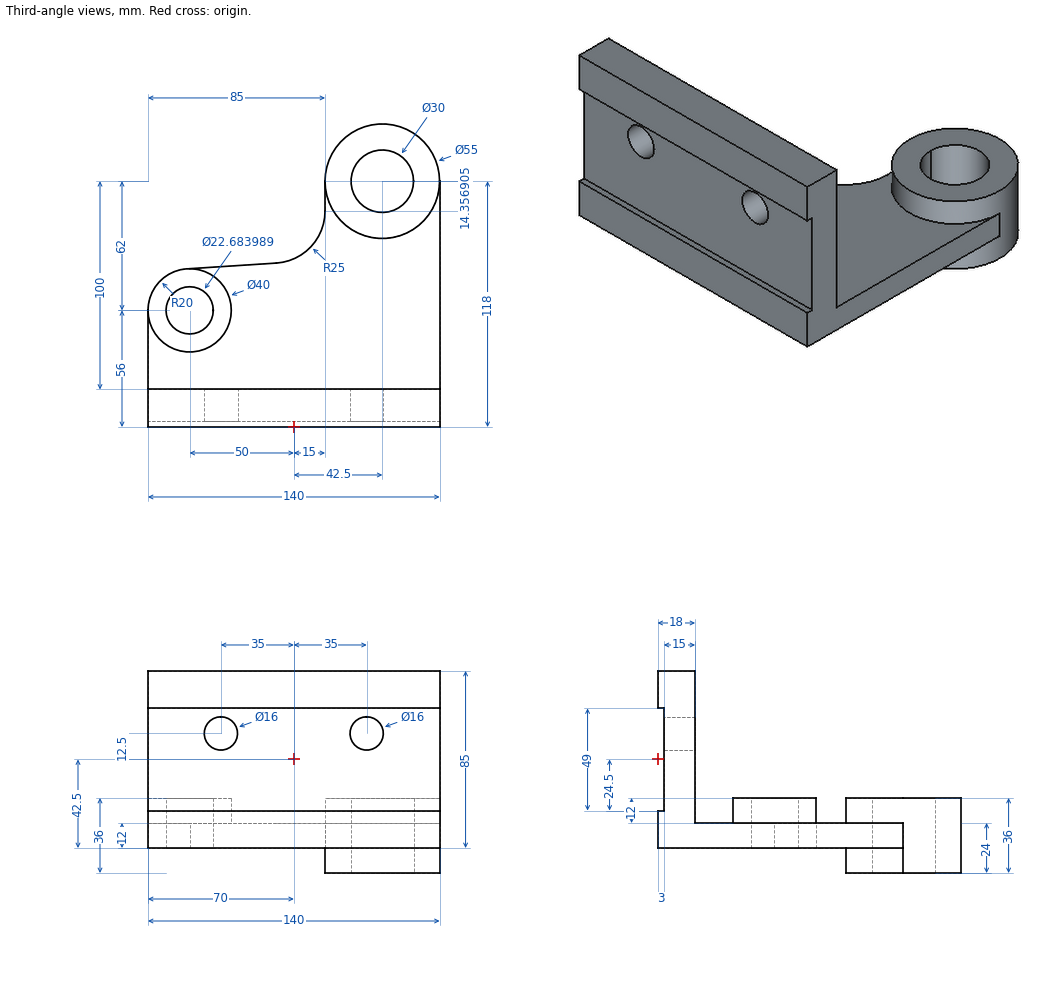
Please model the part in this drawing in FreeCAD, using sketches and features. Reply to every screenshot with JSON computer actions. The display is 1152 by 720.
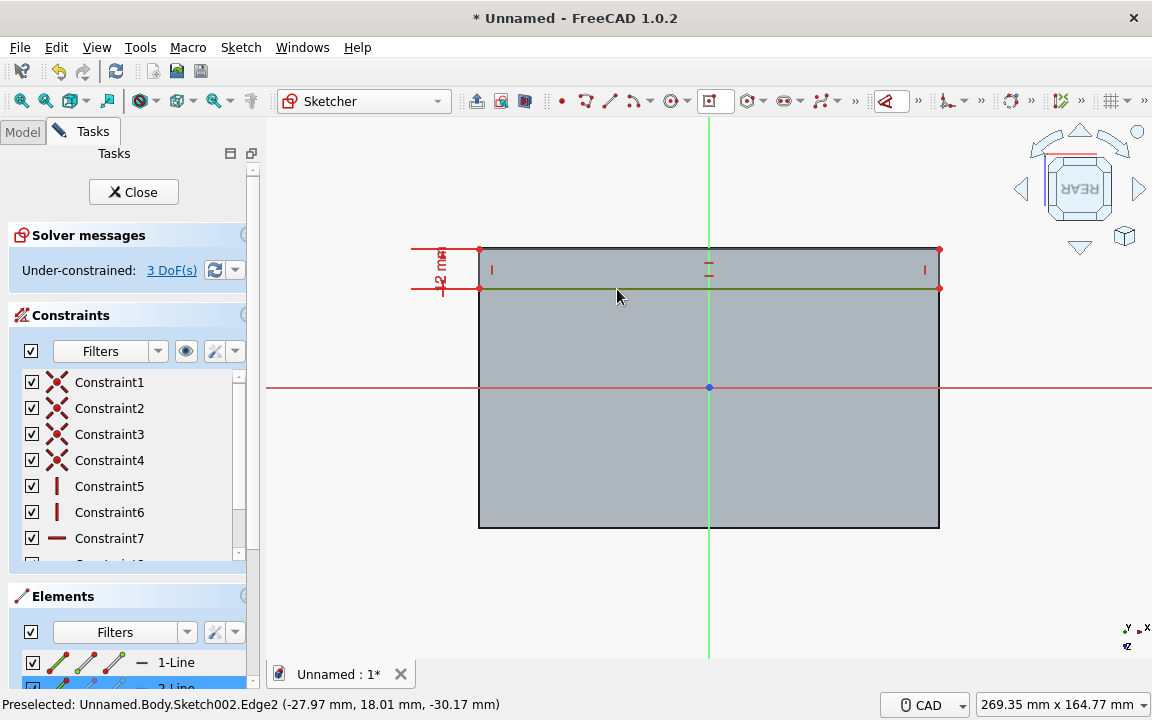
{"action": "key", "text": "l"}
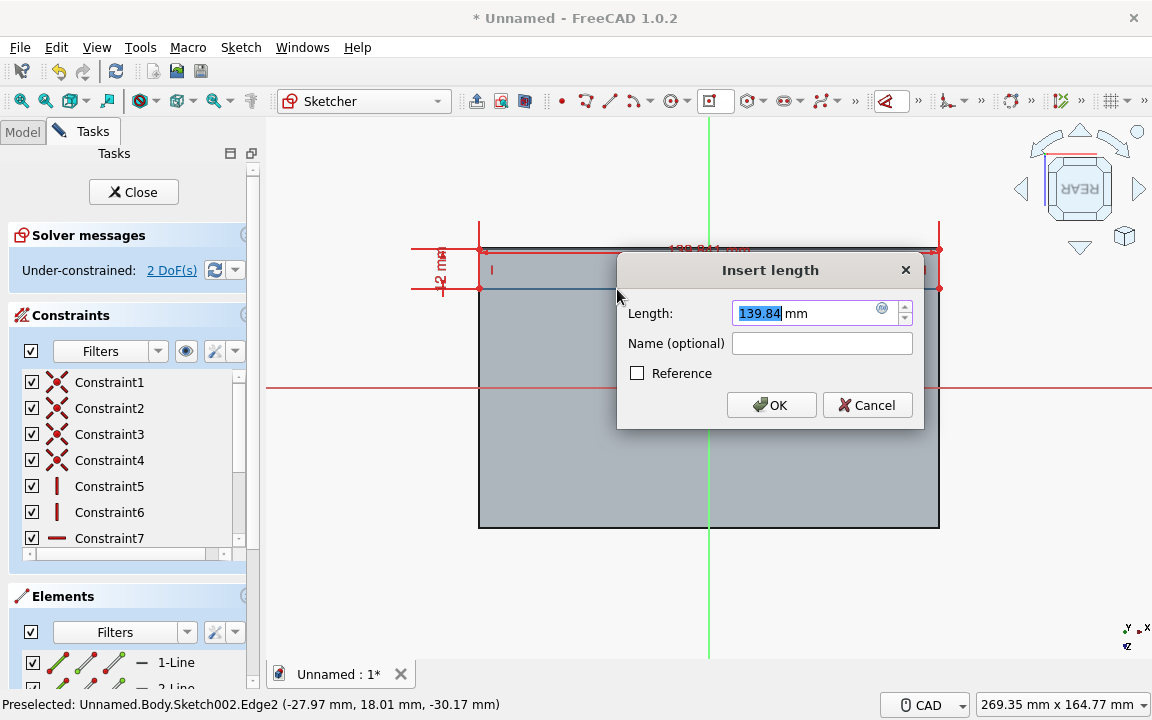
{"action": "type", "text": "140"}
{"action": "key", "text": "Return"}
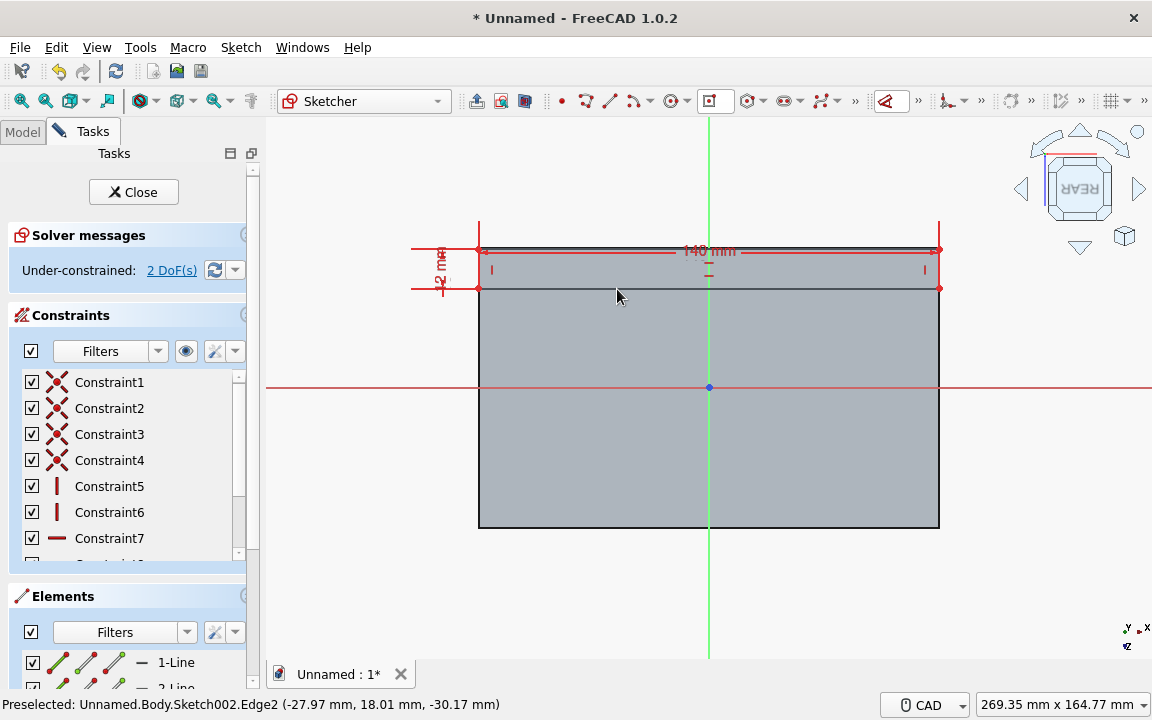
{"action": "left_click", "coordinate": [479, 249]}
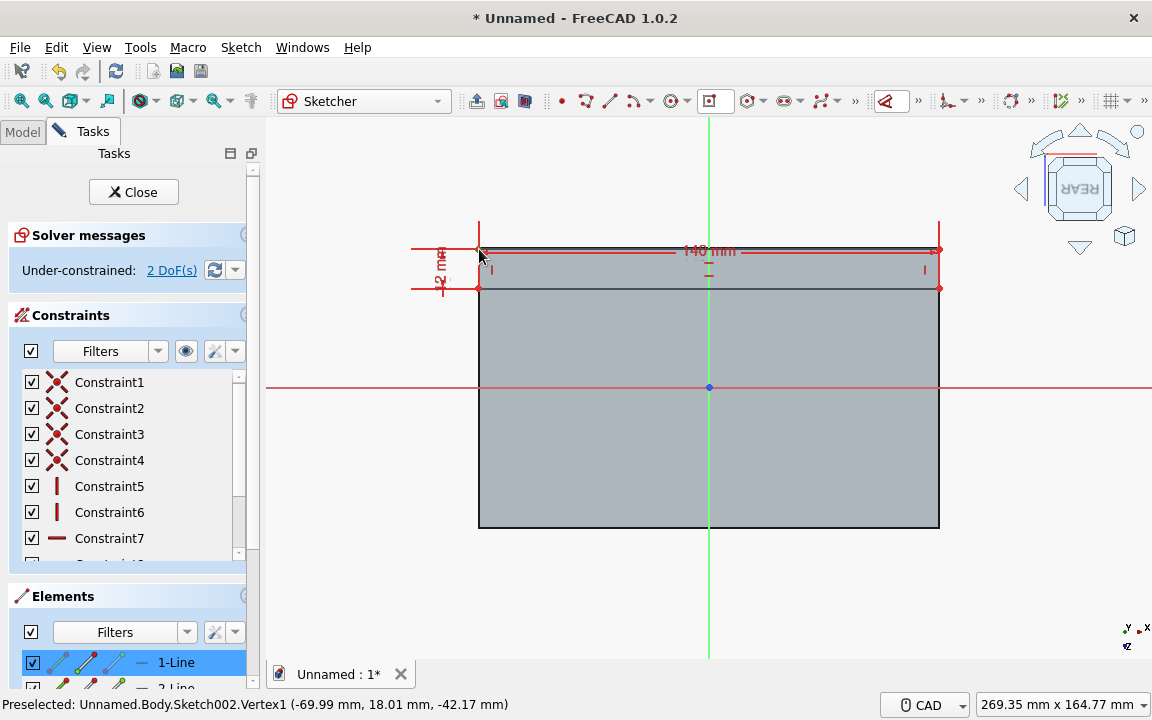
{"action": "key", "text": "l"}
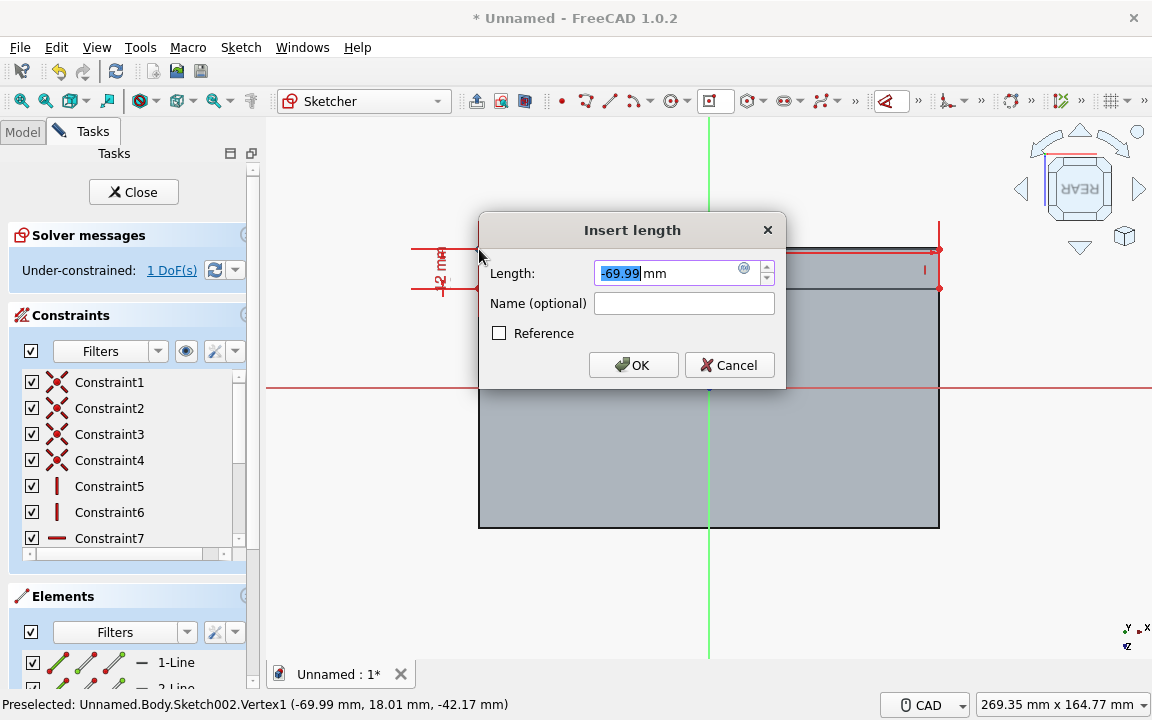
{"action": "type", "text": "-70"}
{"action": "key", "text": "Return"}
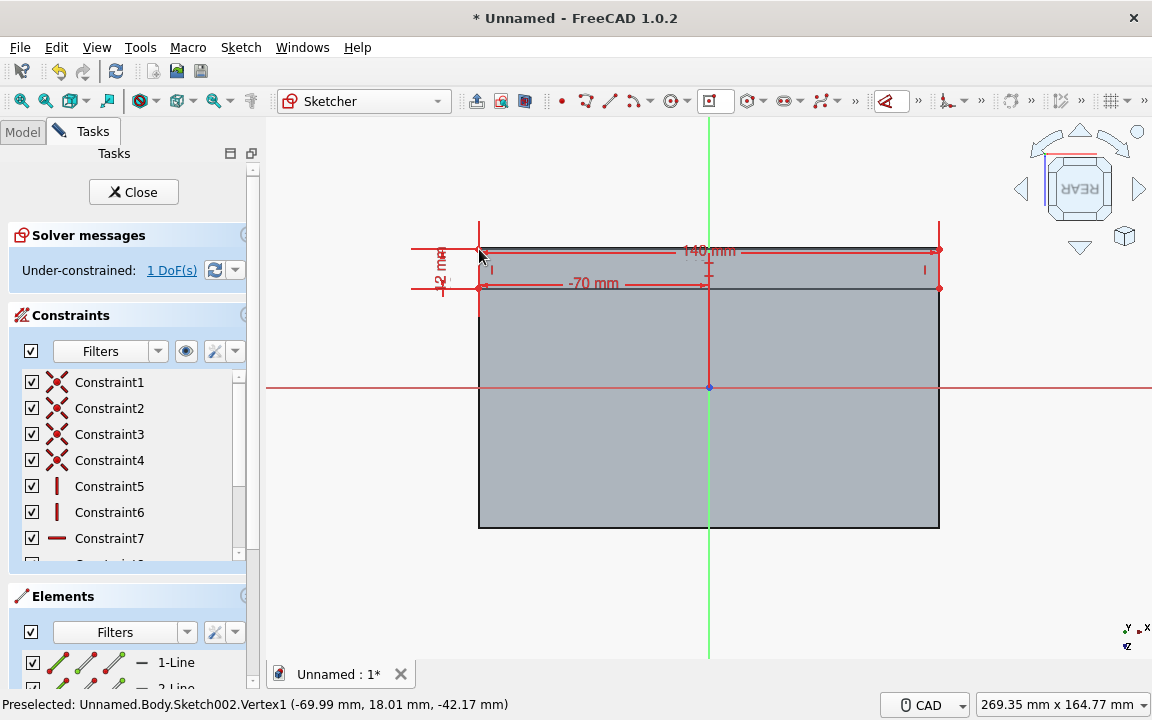
{"action": "left_click", "coordinate": [479, 249]}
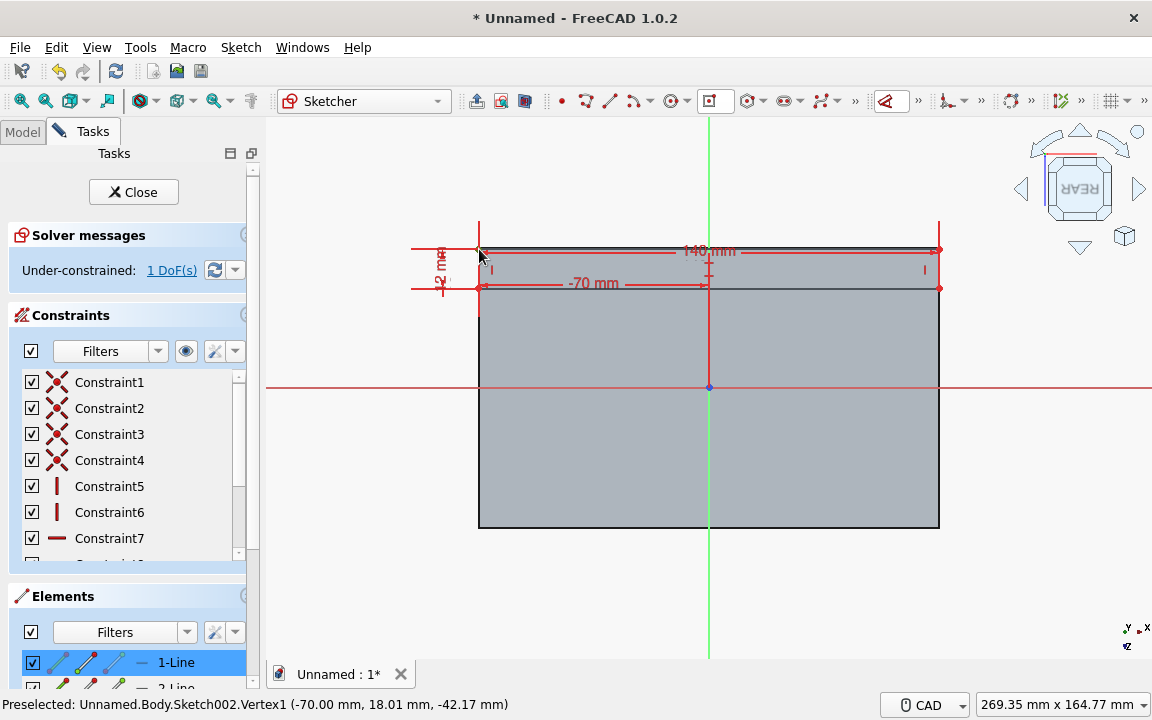
{"action": "key", "text": "i"}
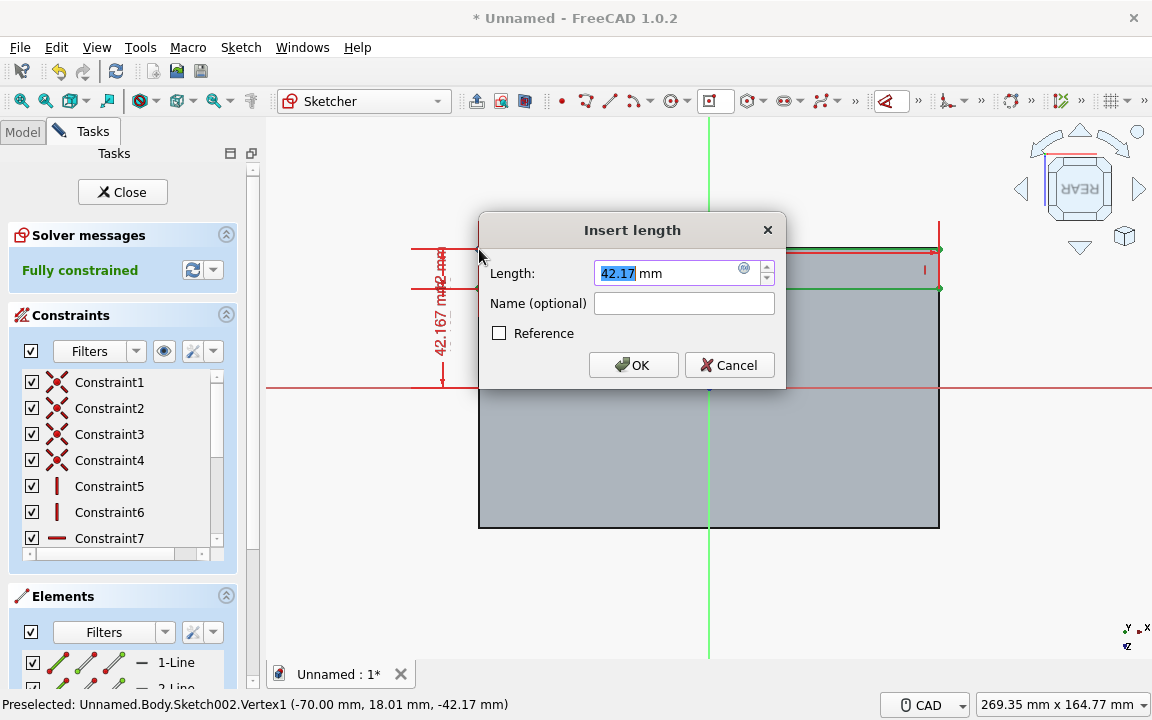
{"action": "type", "text": "42.5"}
{"action": "key", "text": "Return"}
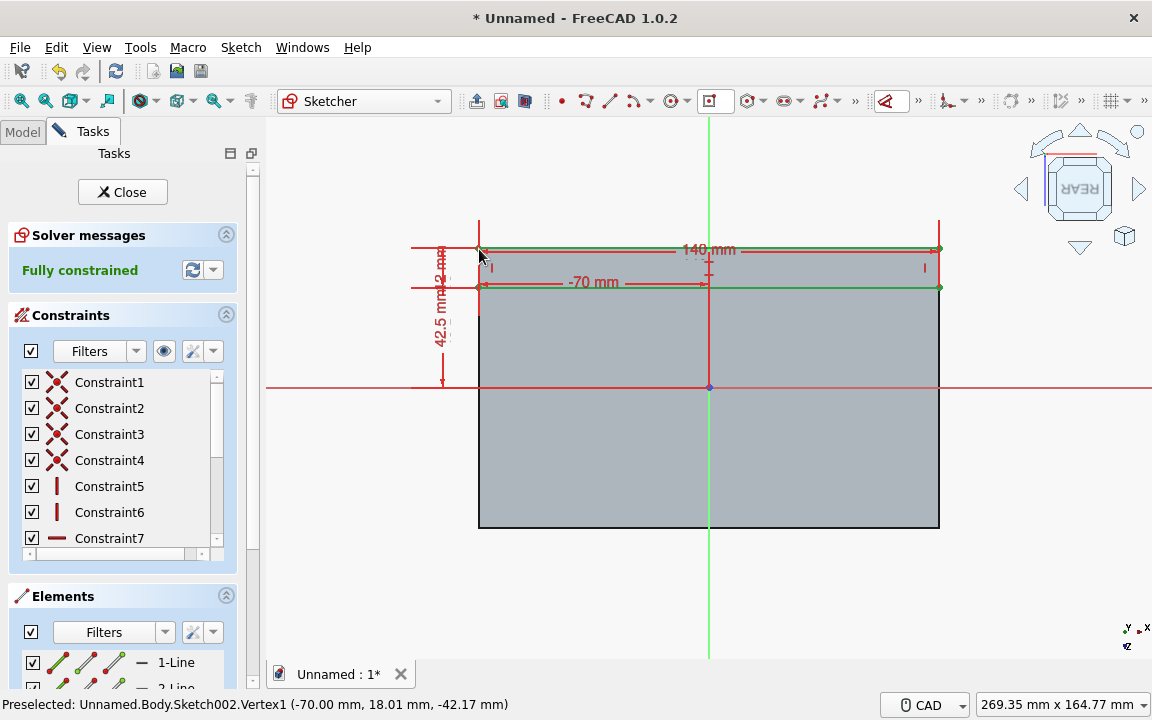
{"action": "left_click", "coordinate": [123, 192]}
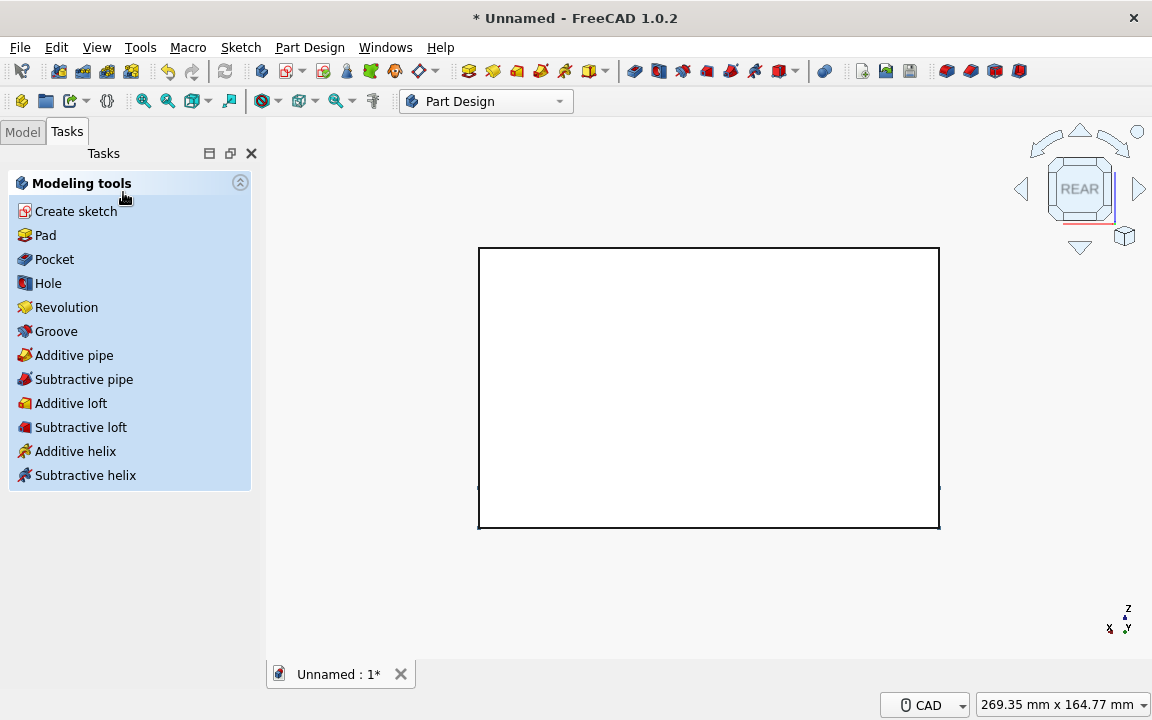
{"action": "left_click", "coordinate": [470, 72]}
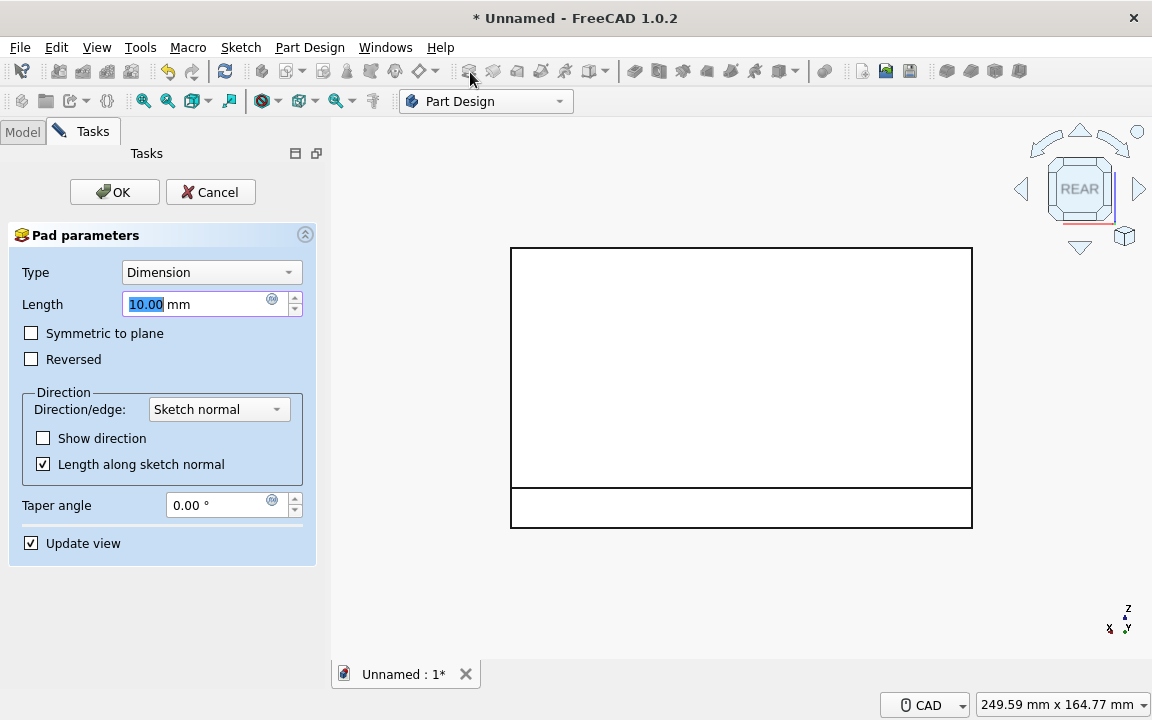
{"action": "type", "text": "100"}
{"action": "key", "text": "Tab"}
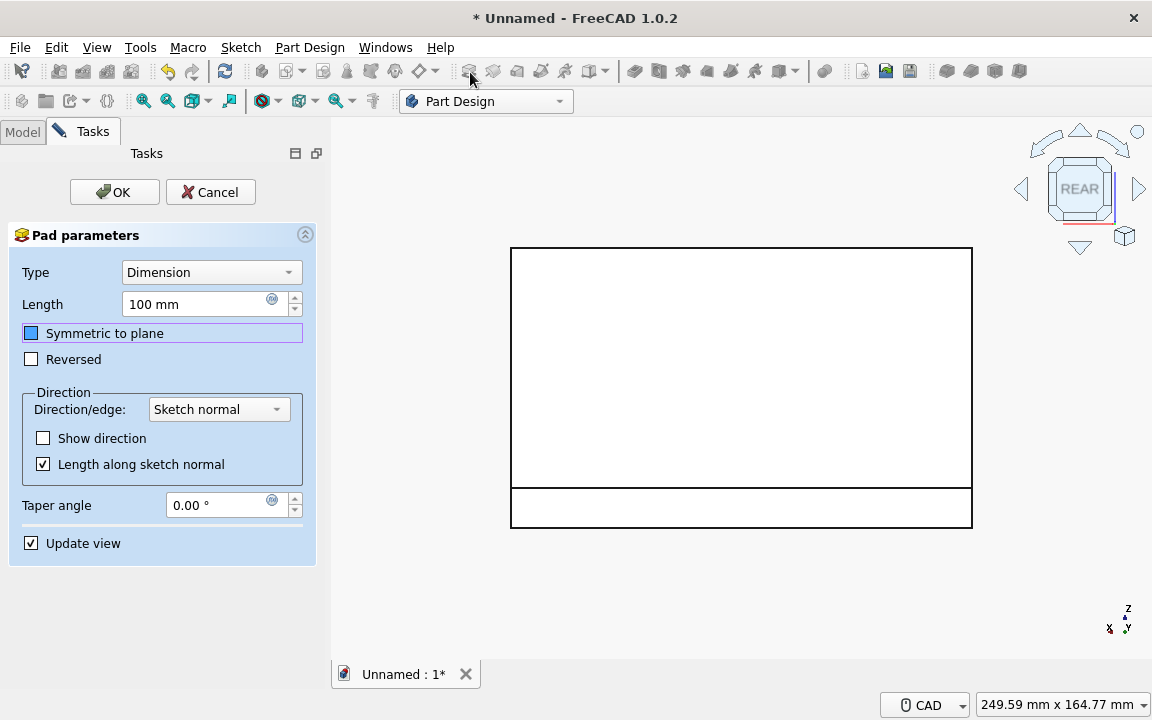
{"action": "left_click", "coordinate": [115, 192]}